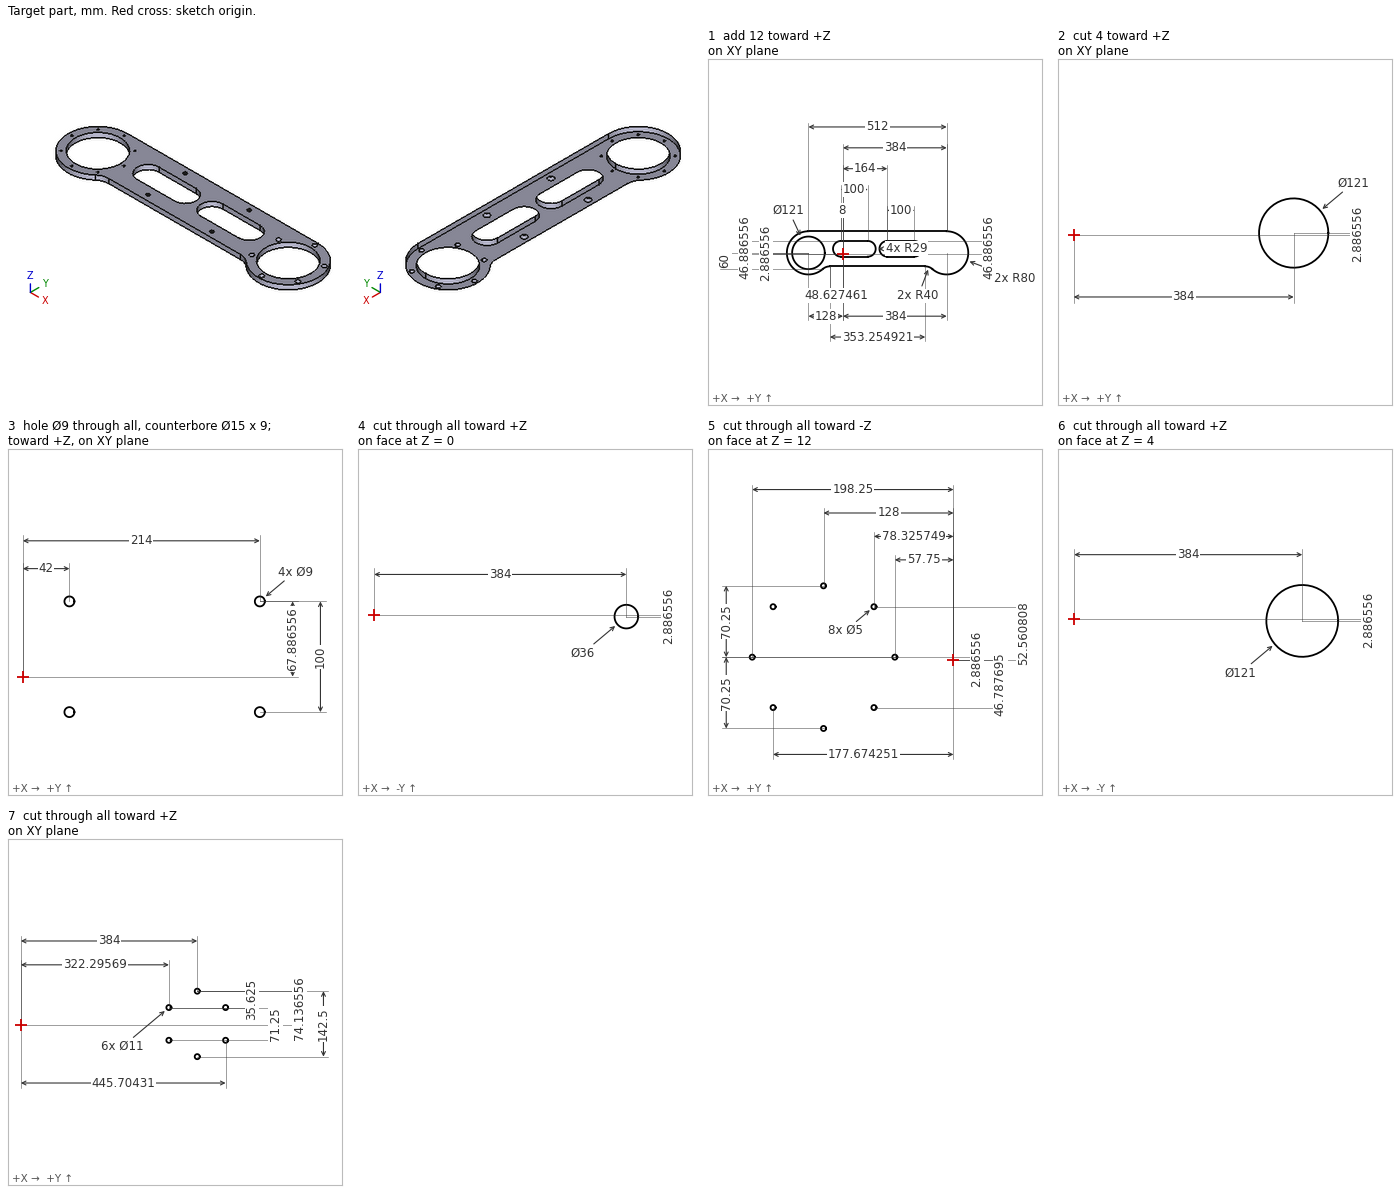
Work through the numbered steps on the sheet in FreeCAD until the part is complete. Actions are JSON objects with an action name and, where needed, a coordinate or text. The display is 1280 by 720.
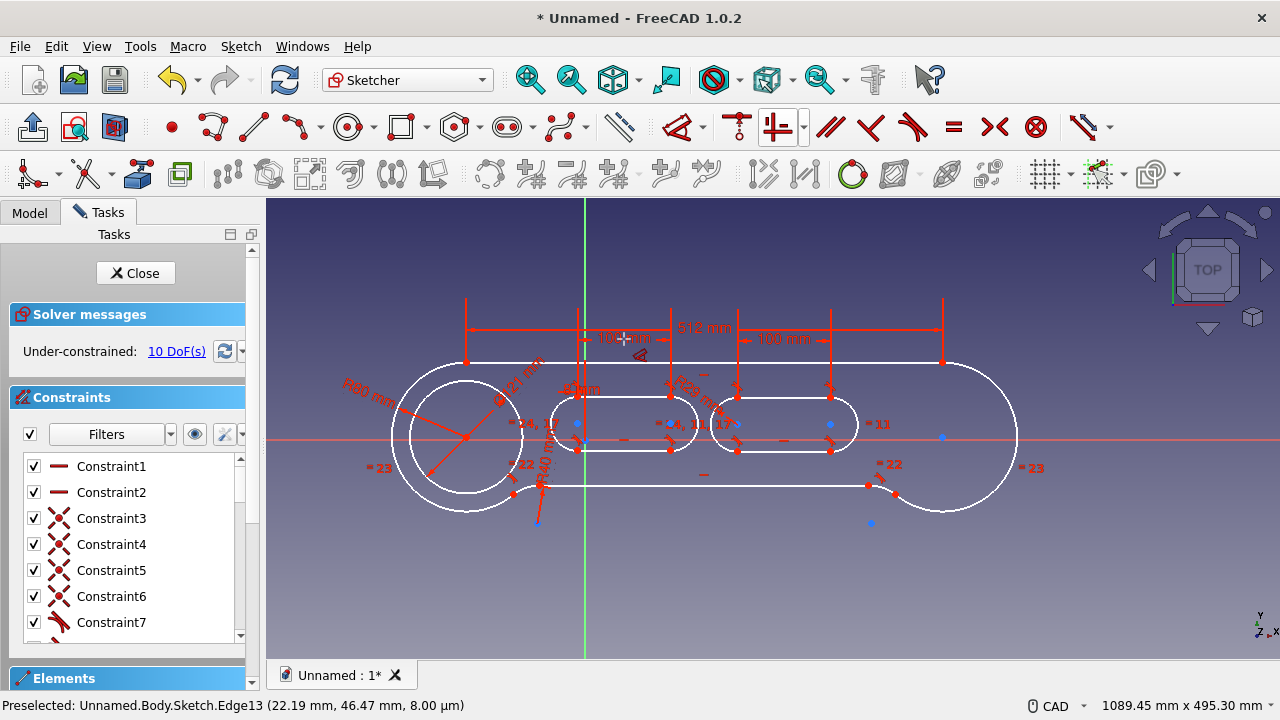
{"action": "left_click", "coordinate": [466, 437]}
{"action": "left_click", "coordinate": [526, 474]}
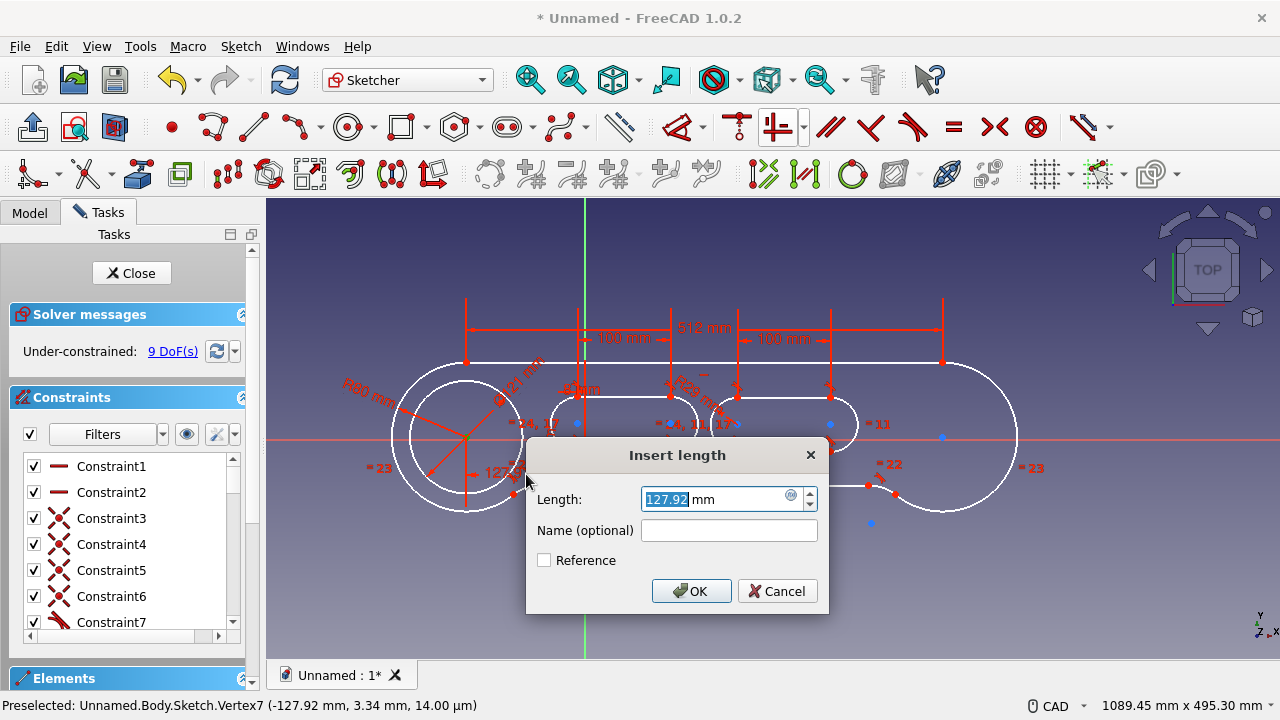
{"action": "type", "text": "128"}
{"action": "key", "text": "Return"}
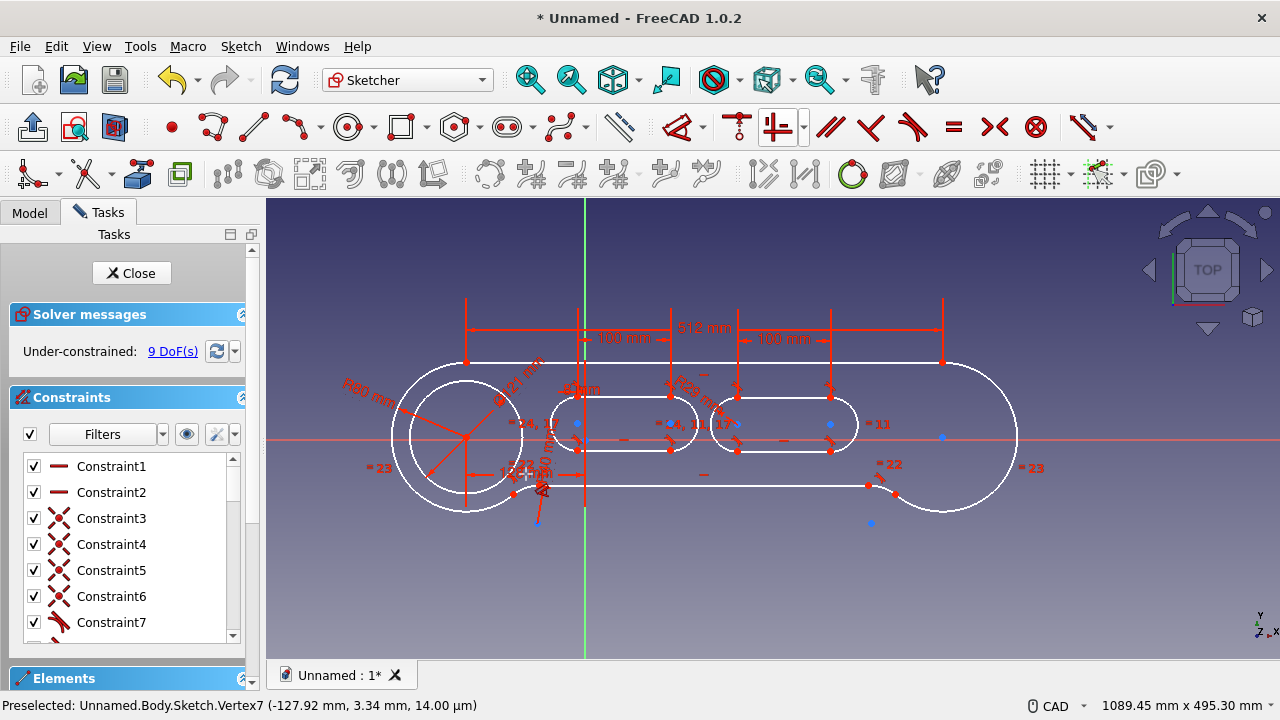
{"action": "left_click", "coordinate": [514, 494]}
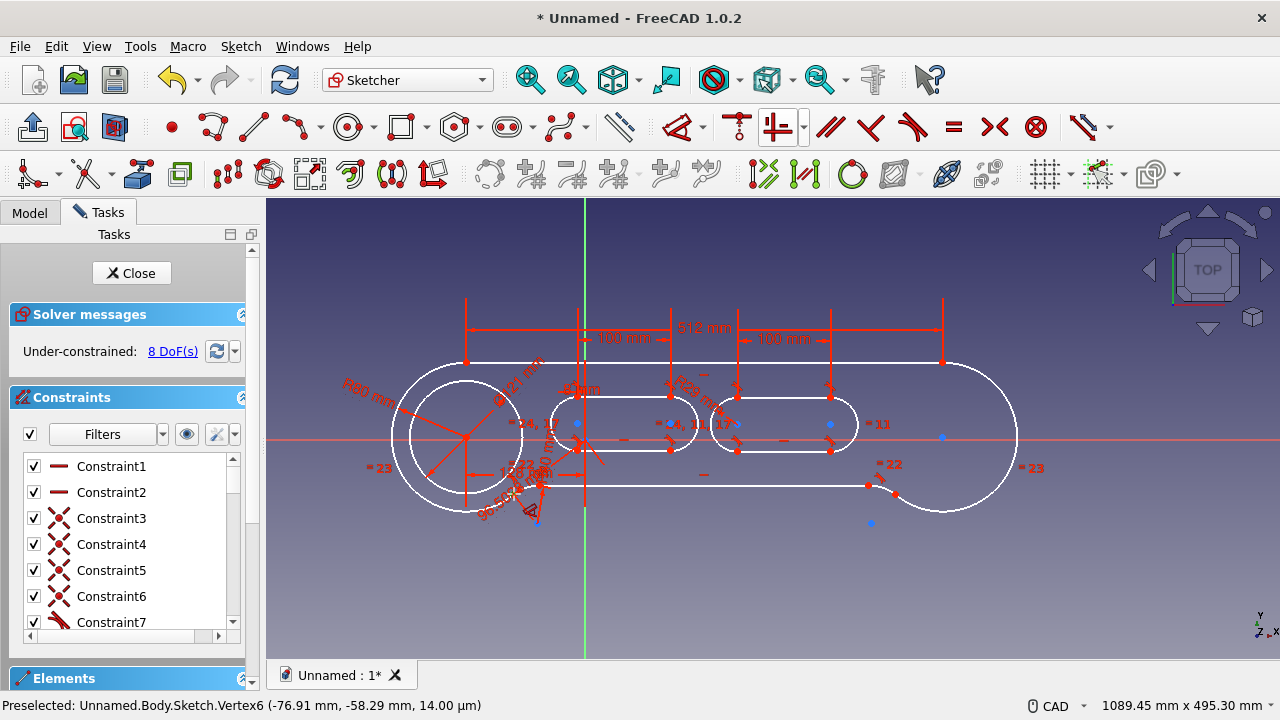
{"action": "left_click", "coordinate": [466, 437]}
{"action": "left_click", "coordinate": [384, 479]}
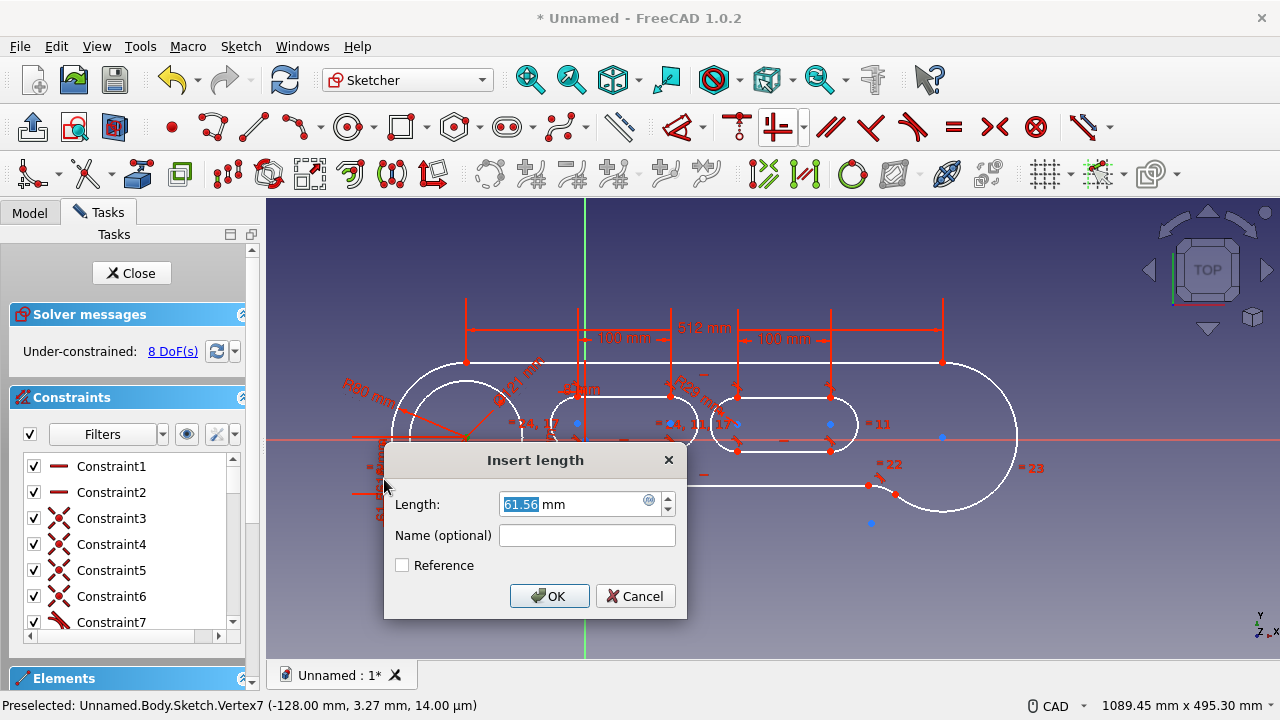
{"action": "type", "text": "60"}
{"action": "key", "text": "Return"}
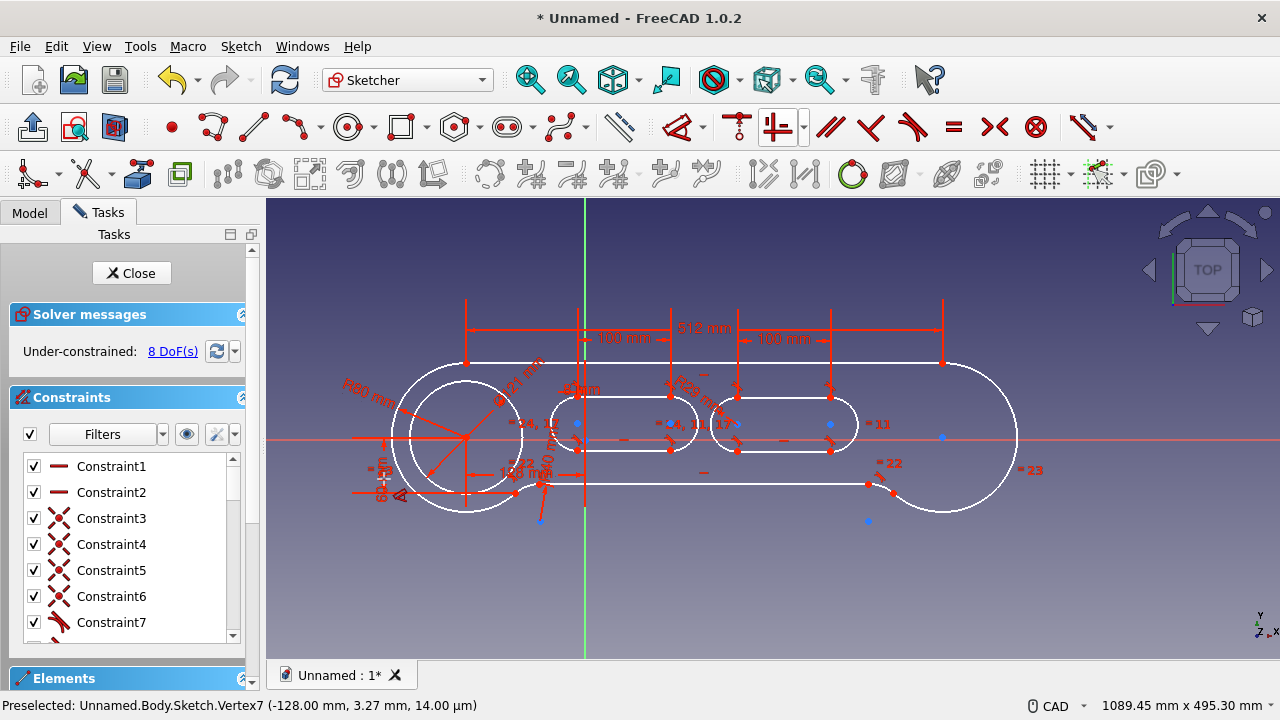
{"action": "left_click", "coordinate": [943, 363]}
{"action": "left_click", "coordinate": [889, 329]}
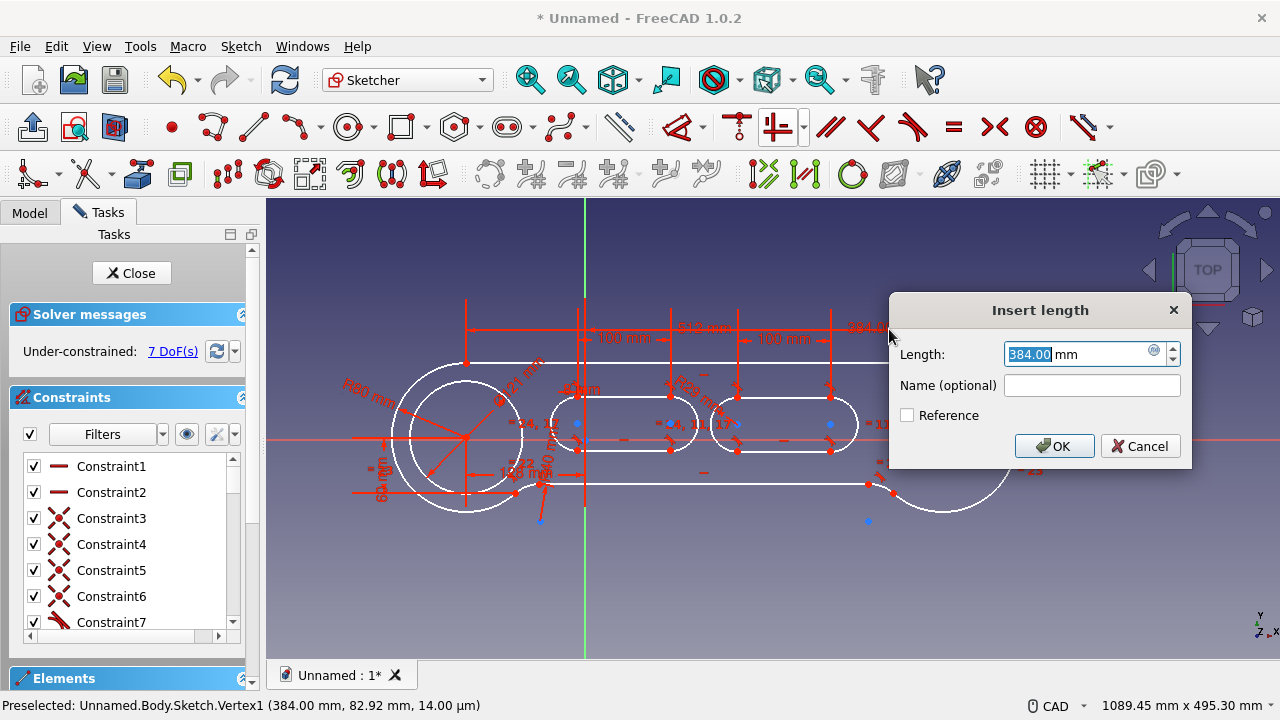
{"action": "type", "text": "384"}
{"action": "key", "text": "Return"}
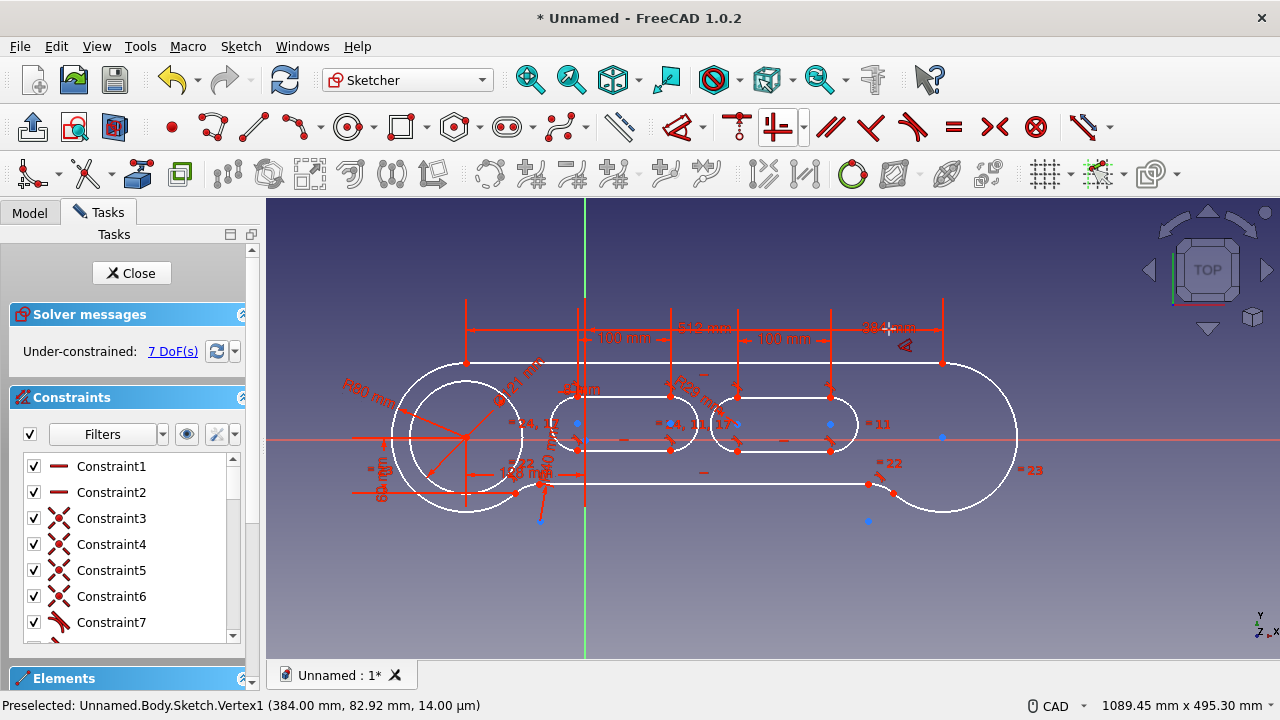
{"action": "left_click", "coordinate": [738, 398]}
{"action": "left_click", "coordinate": [662, 498]}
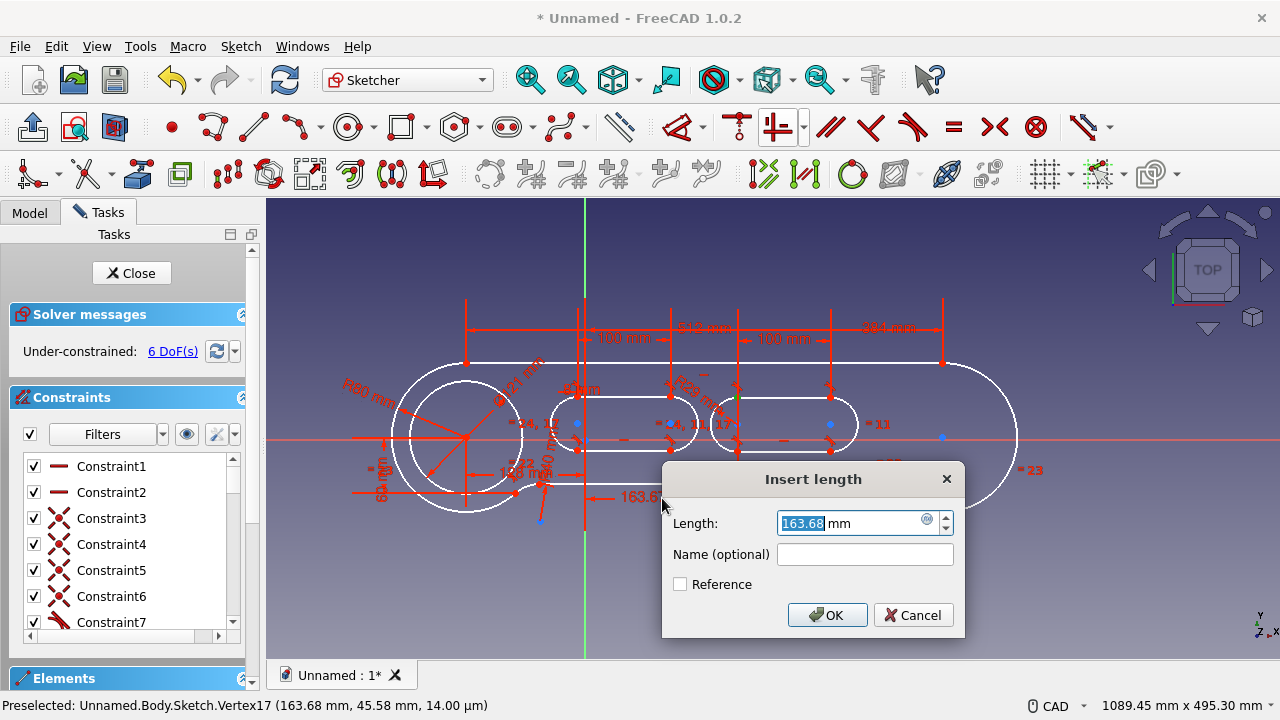
{"action": "type", "text": "164"}
{"action": "key", "text": "Return"}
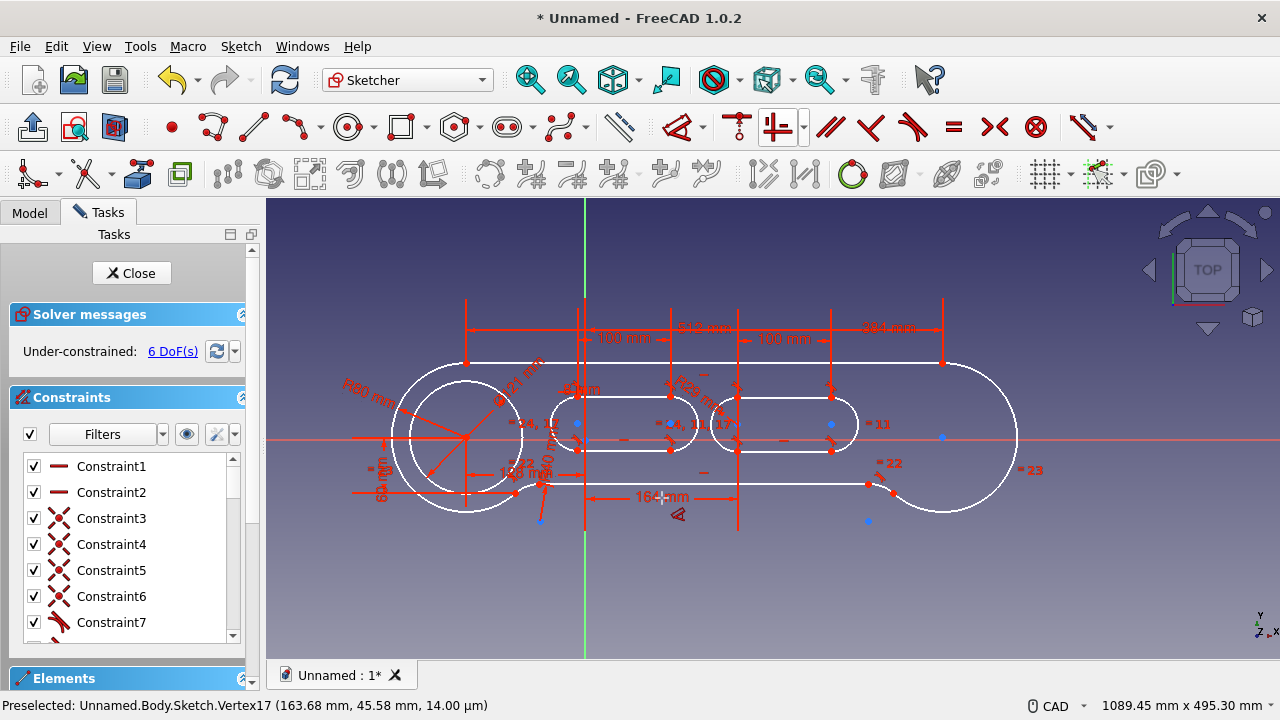
{"action": "left_click", "coordinate": [943, 438]}
{"action": "left_click", "coordinate": [889, 474]}